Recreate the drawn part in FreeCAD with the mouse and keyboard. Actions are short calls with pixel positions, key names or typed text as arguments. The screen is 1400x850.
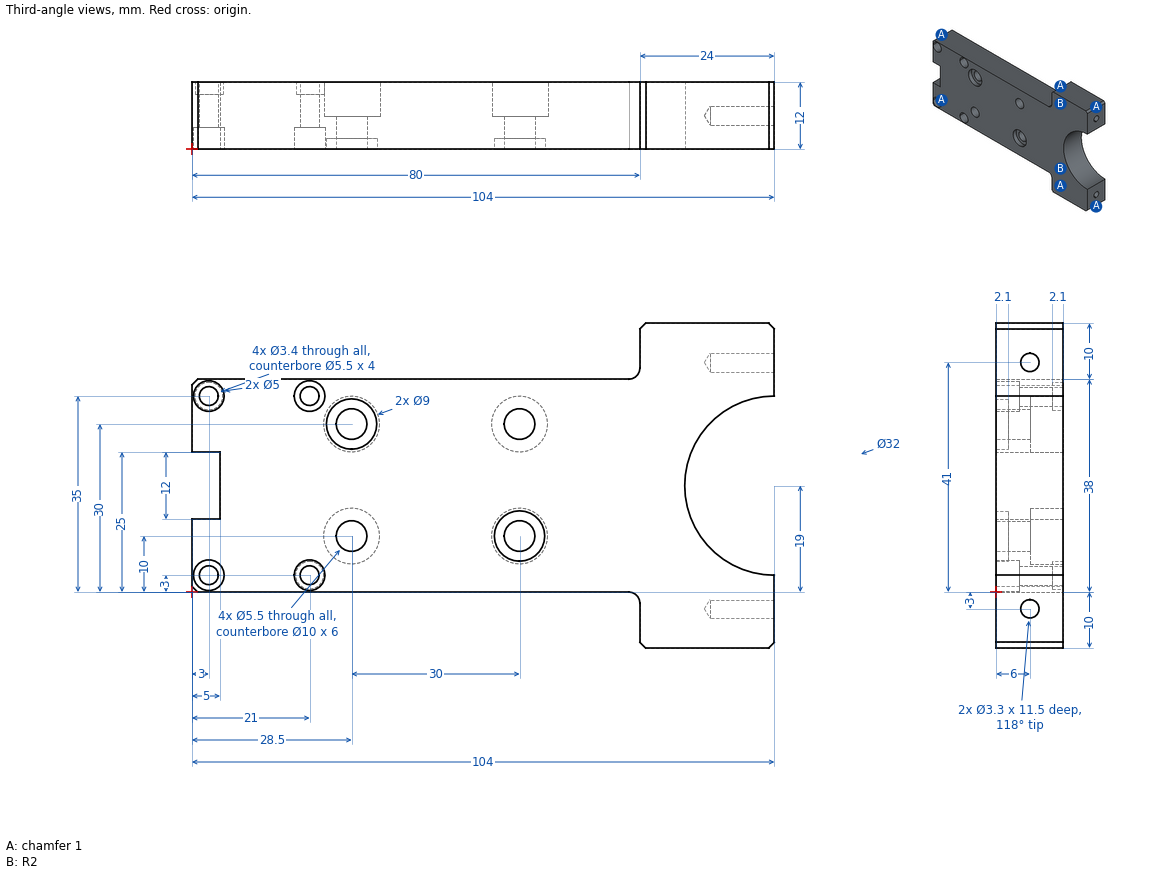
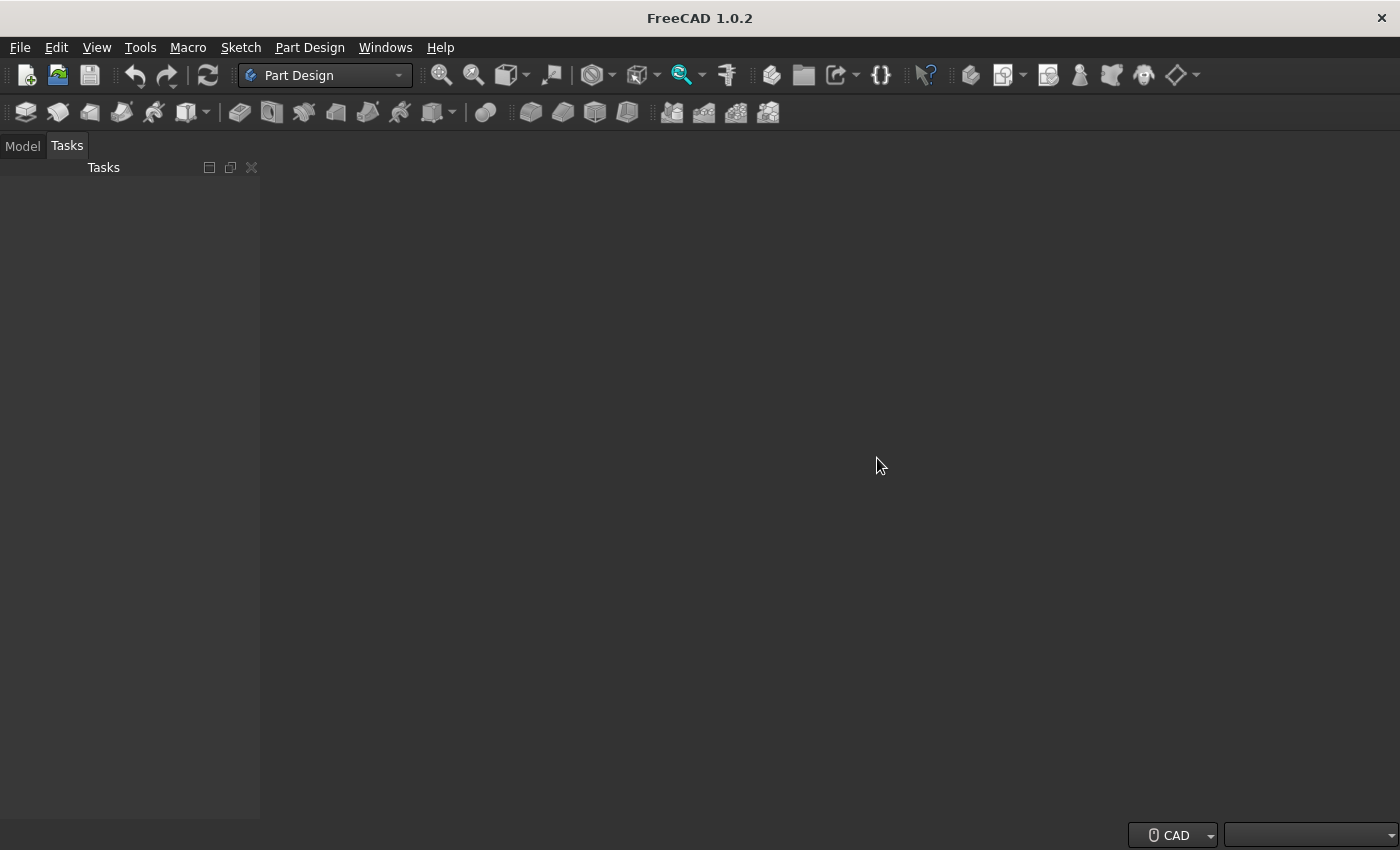
click(26, 76)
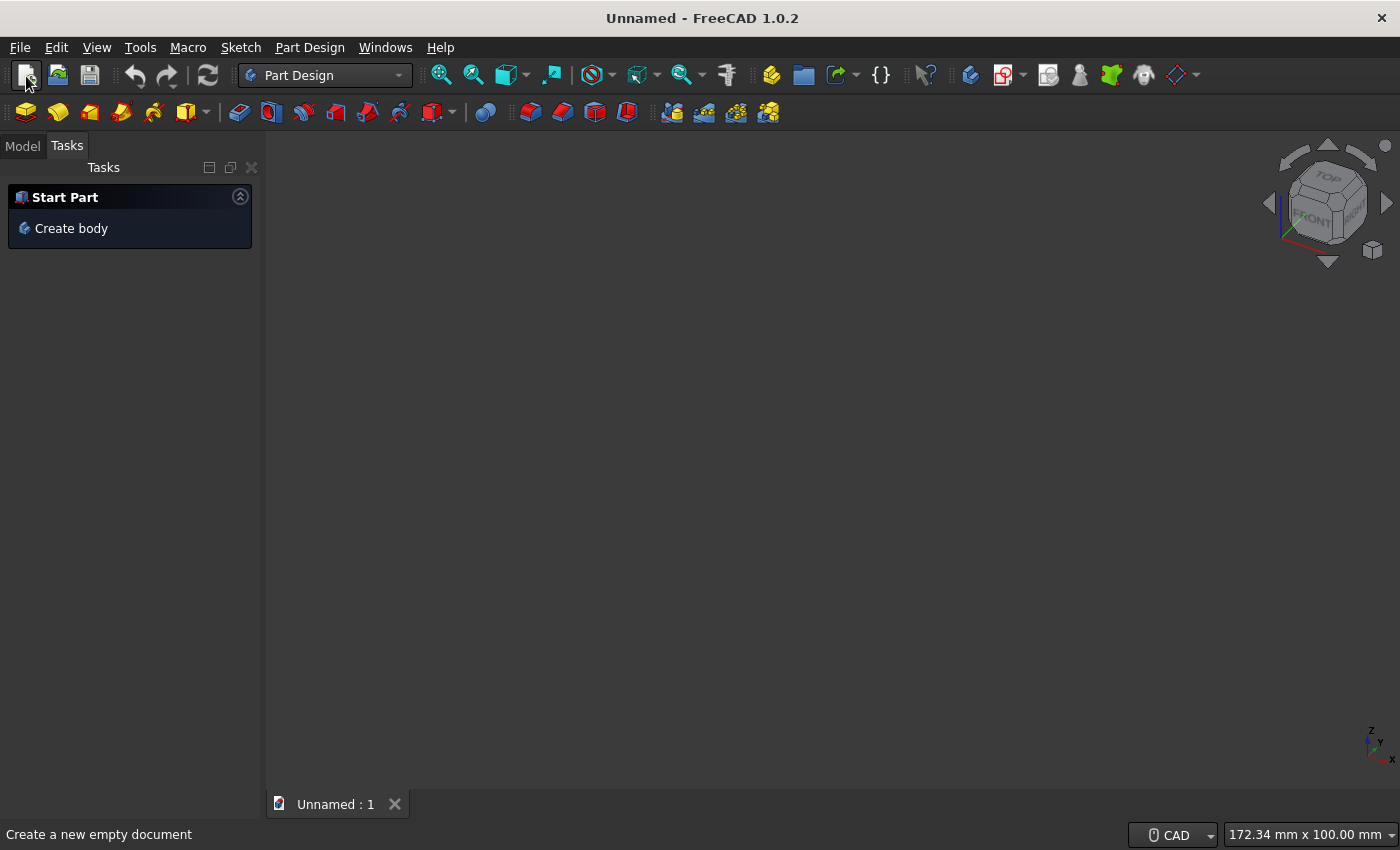
click(1004, 76)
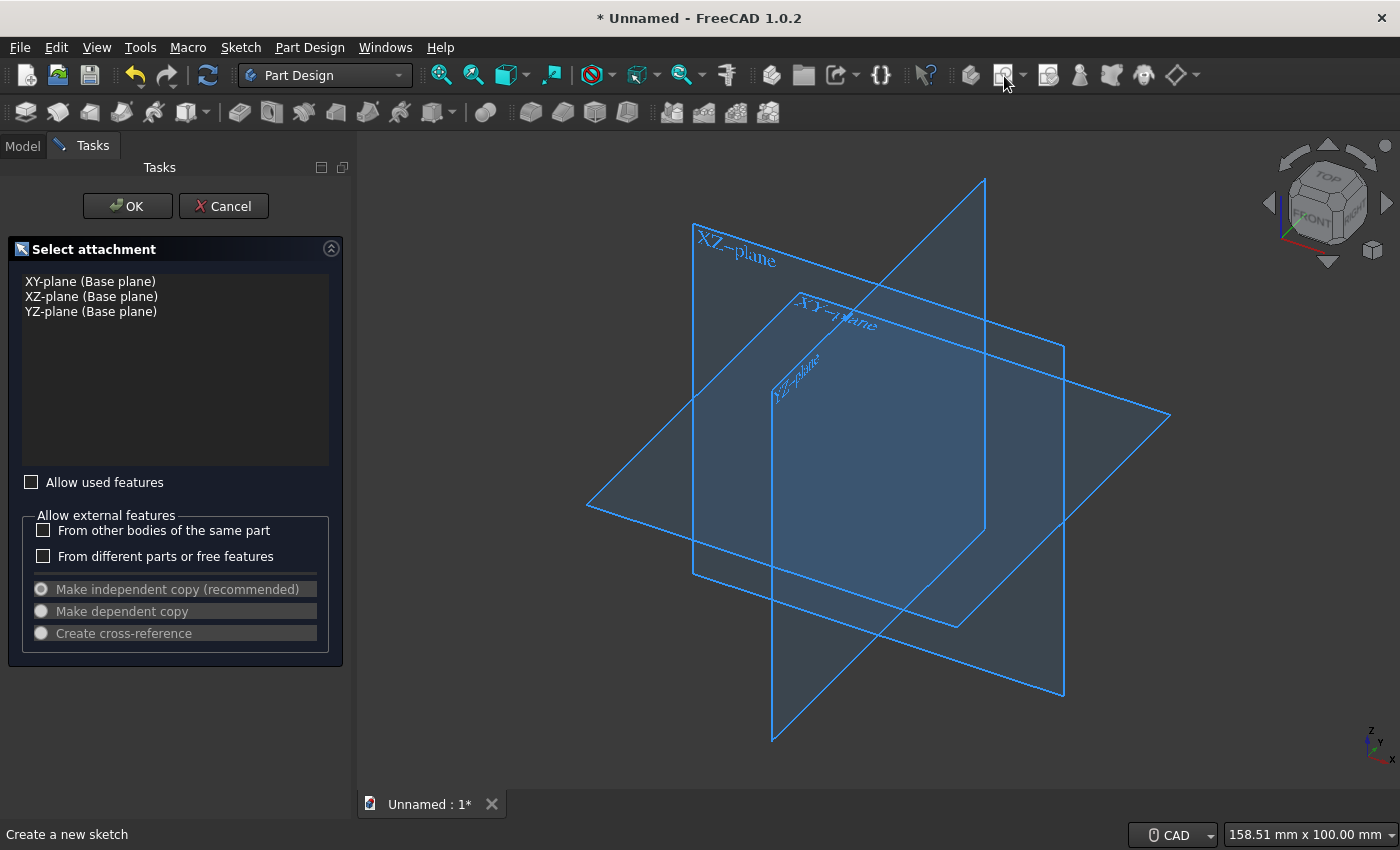
click(82, 282)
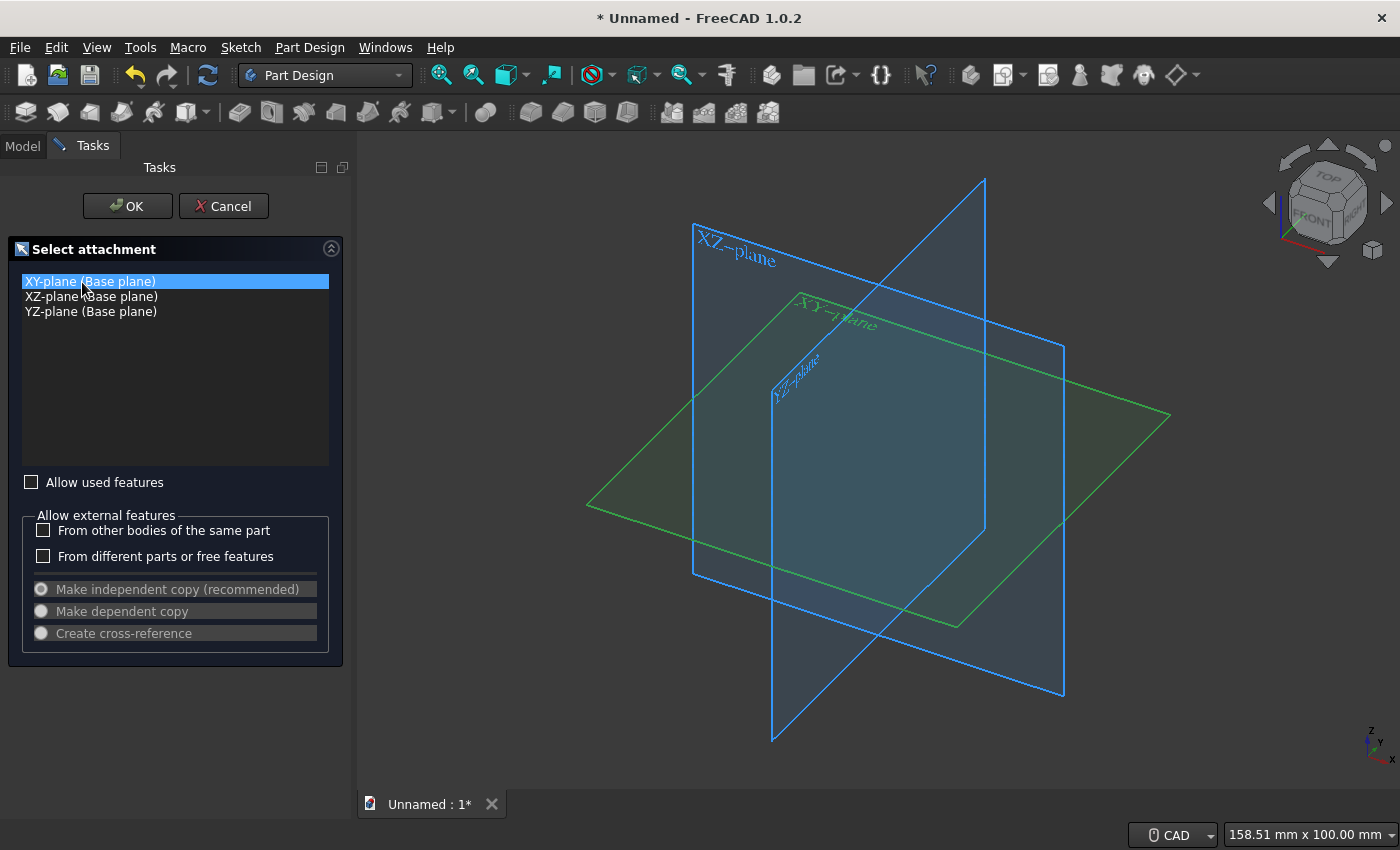
click(128, 206)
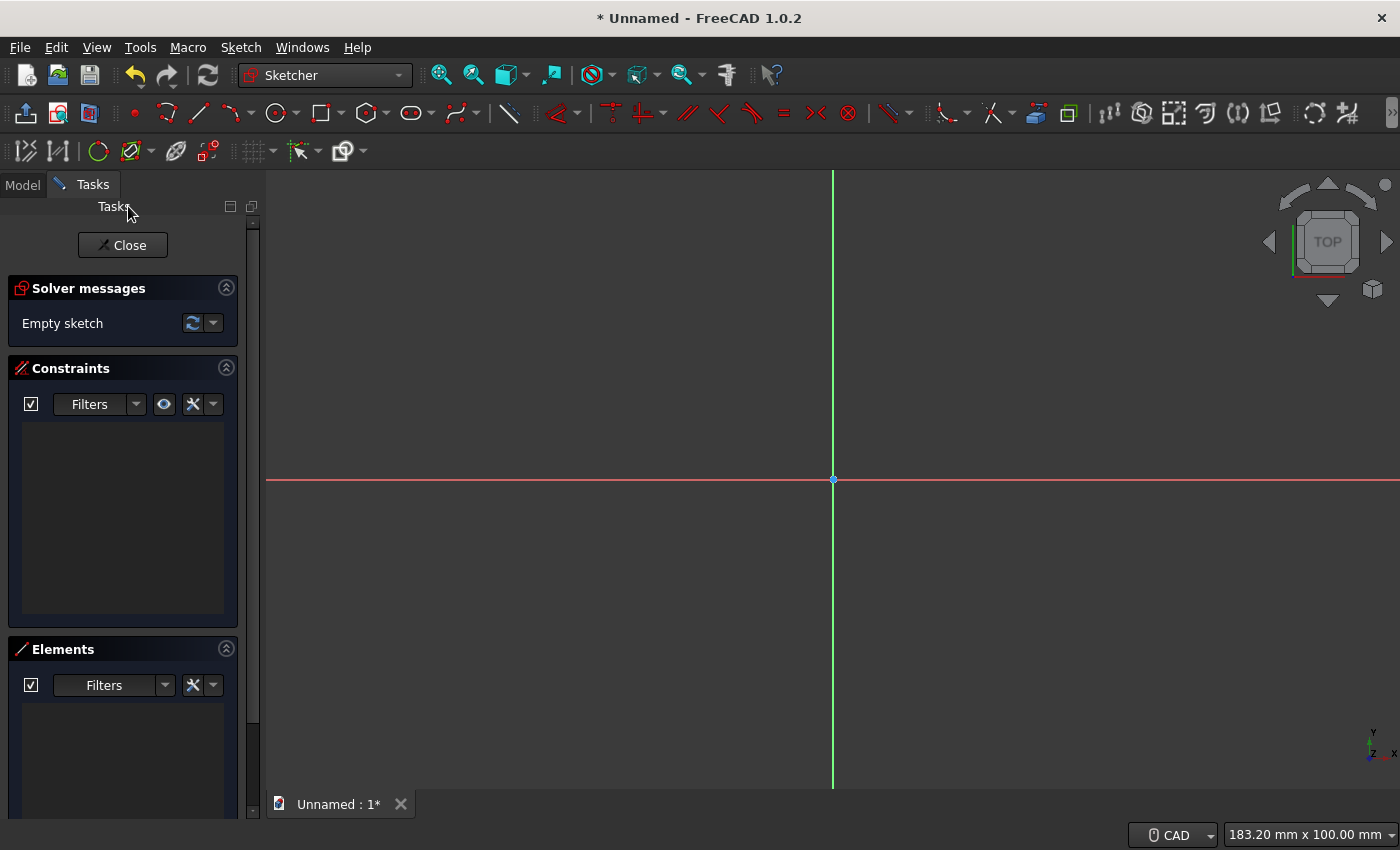
scroll(294, 555, down, 2)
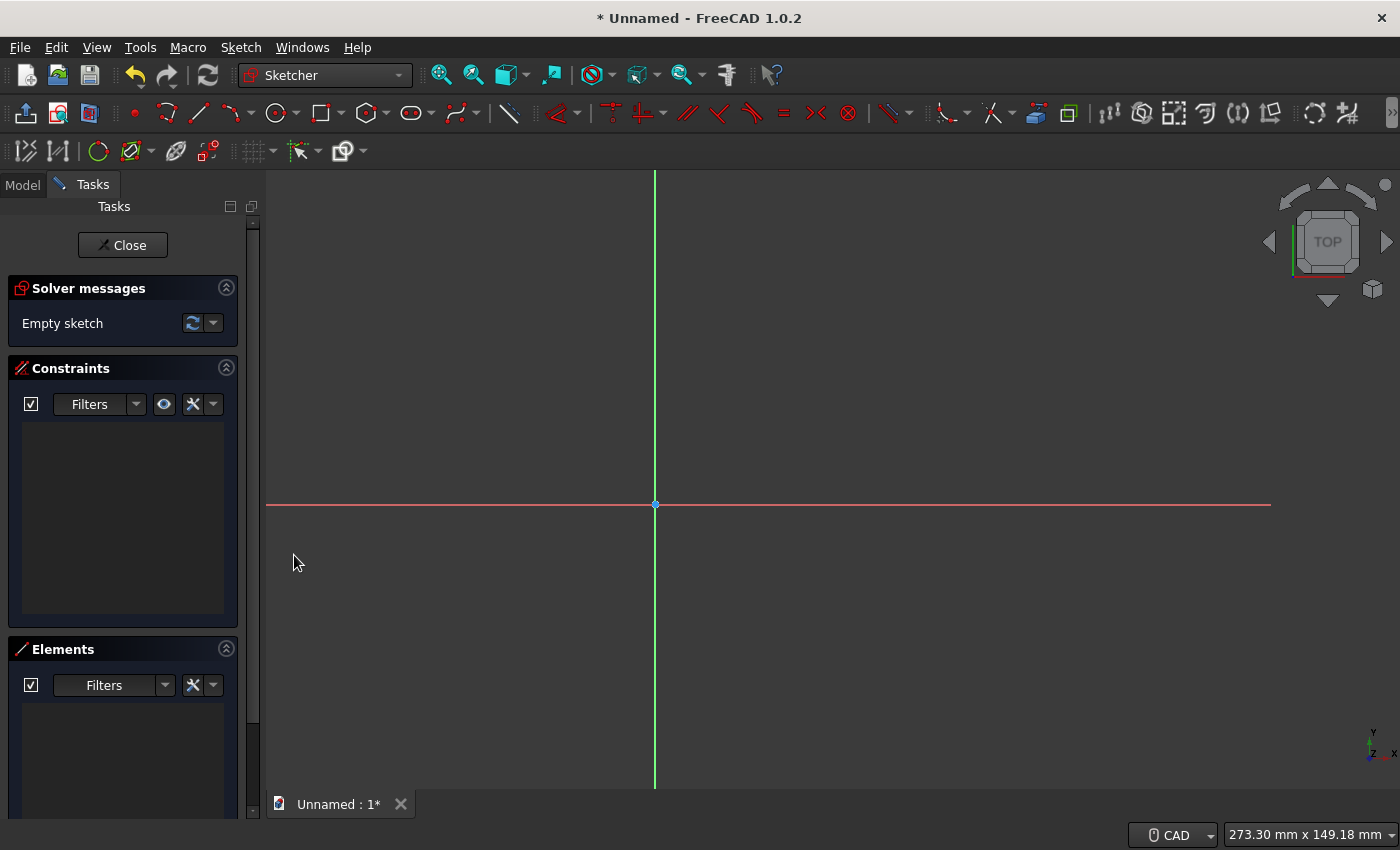
scroll(1088, 480, up, 2)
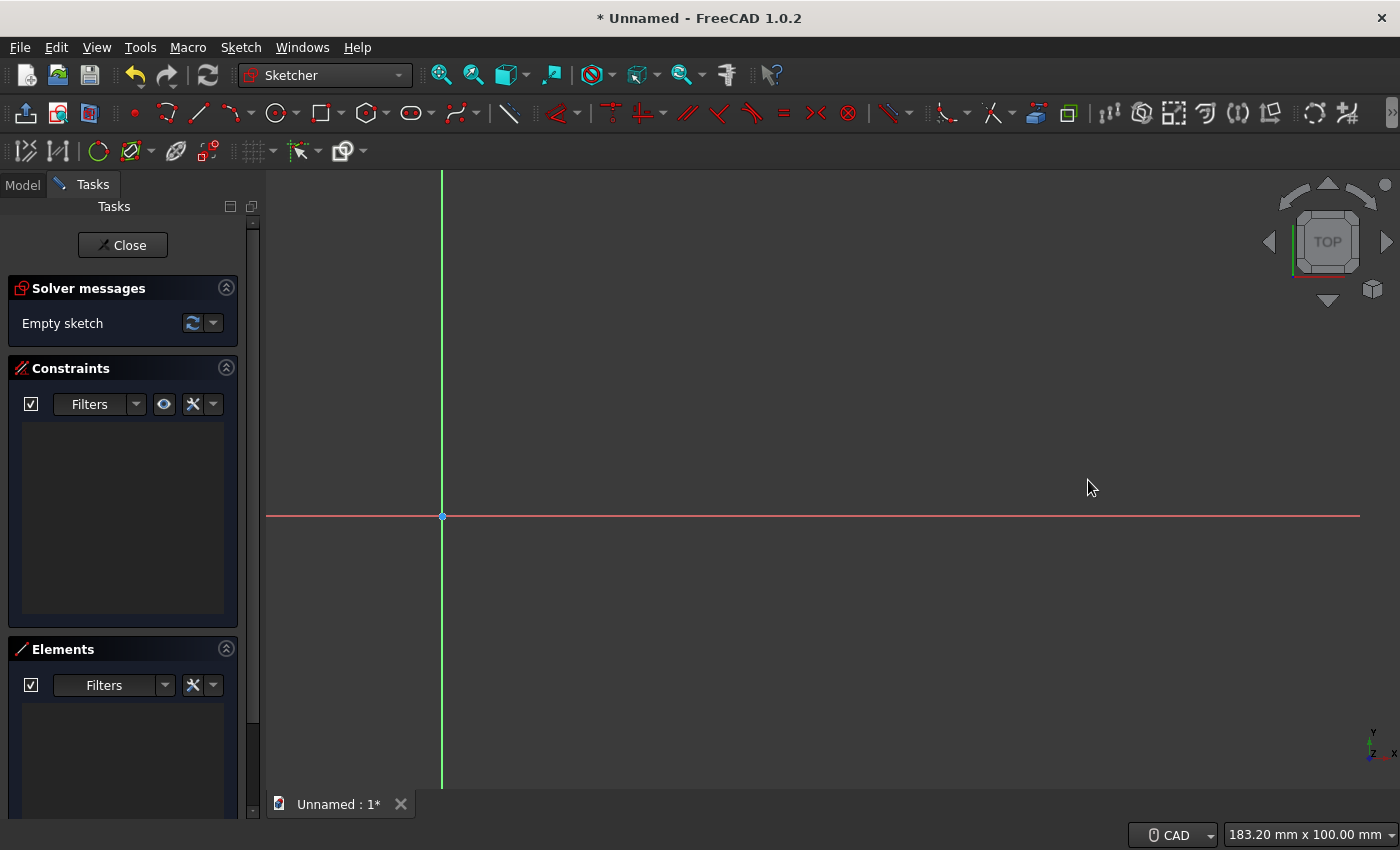
click(322, 114)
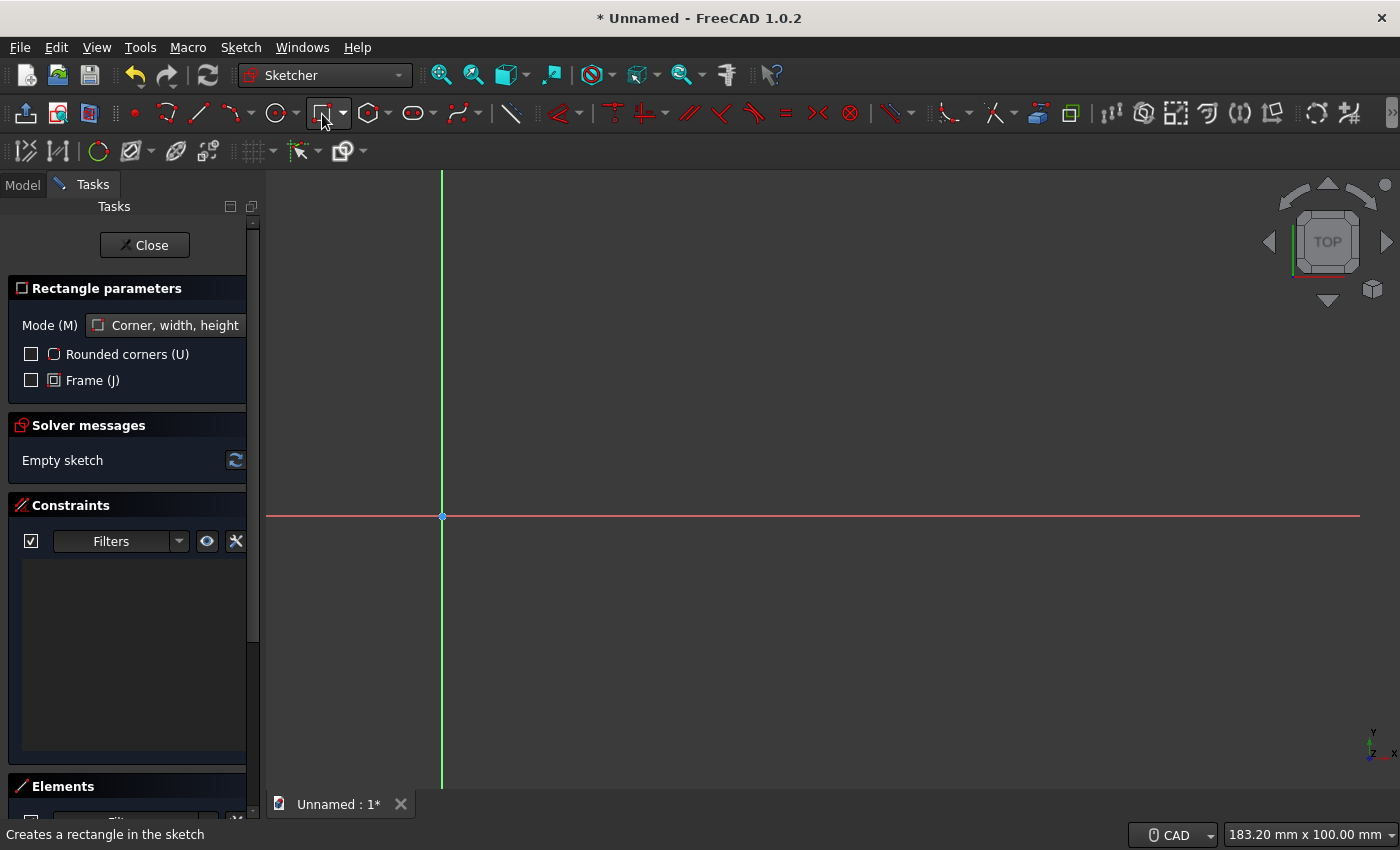
click(442, 516)
click(1086, 442)
key(Escape)